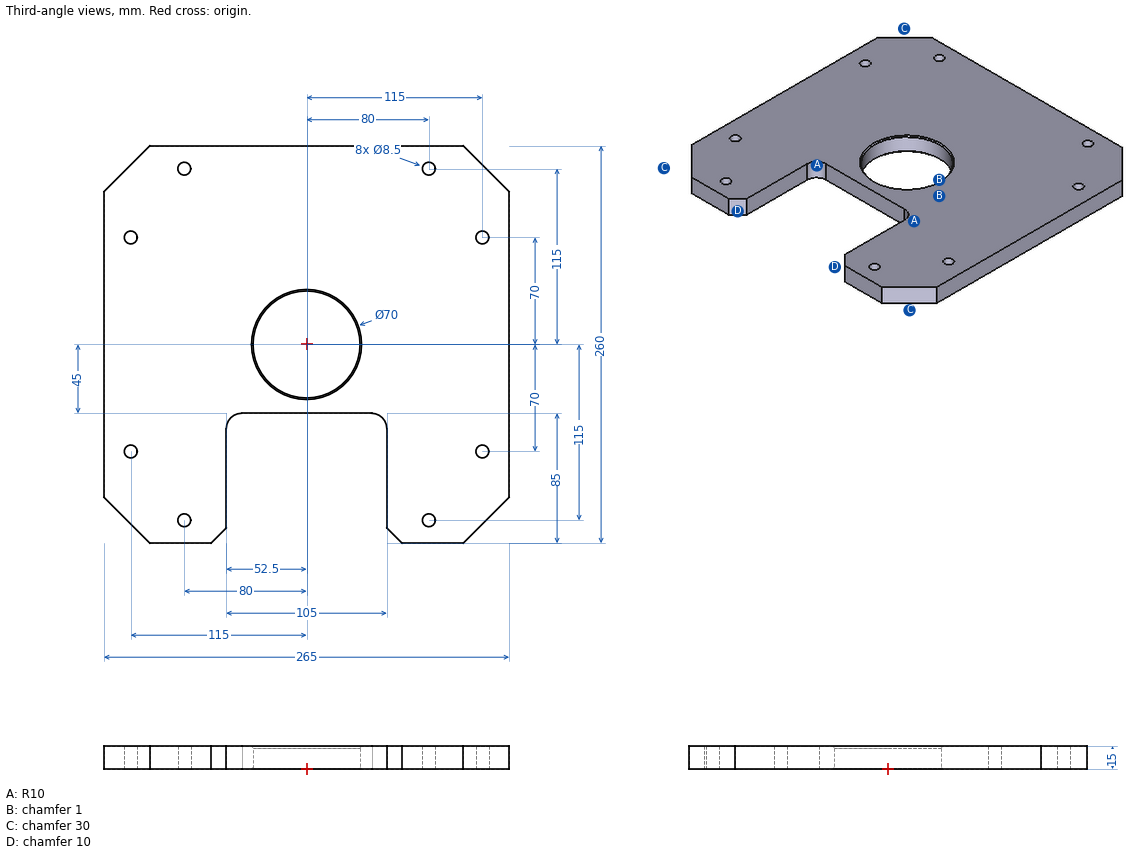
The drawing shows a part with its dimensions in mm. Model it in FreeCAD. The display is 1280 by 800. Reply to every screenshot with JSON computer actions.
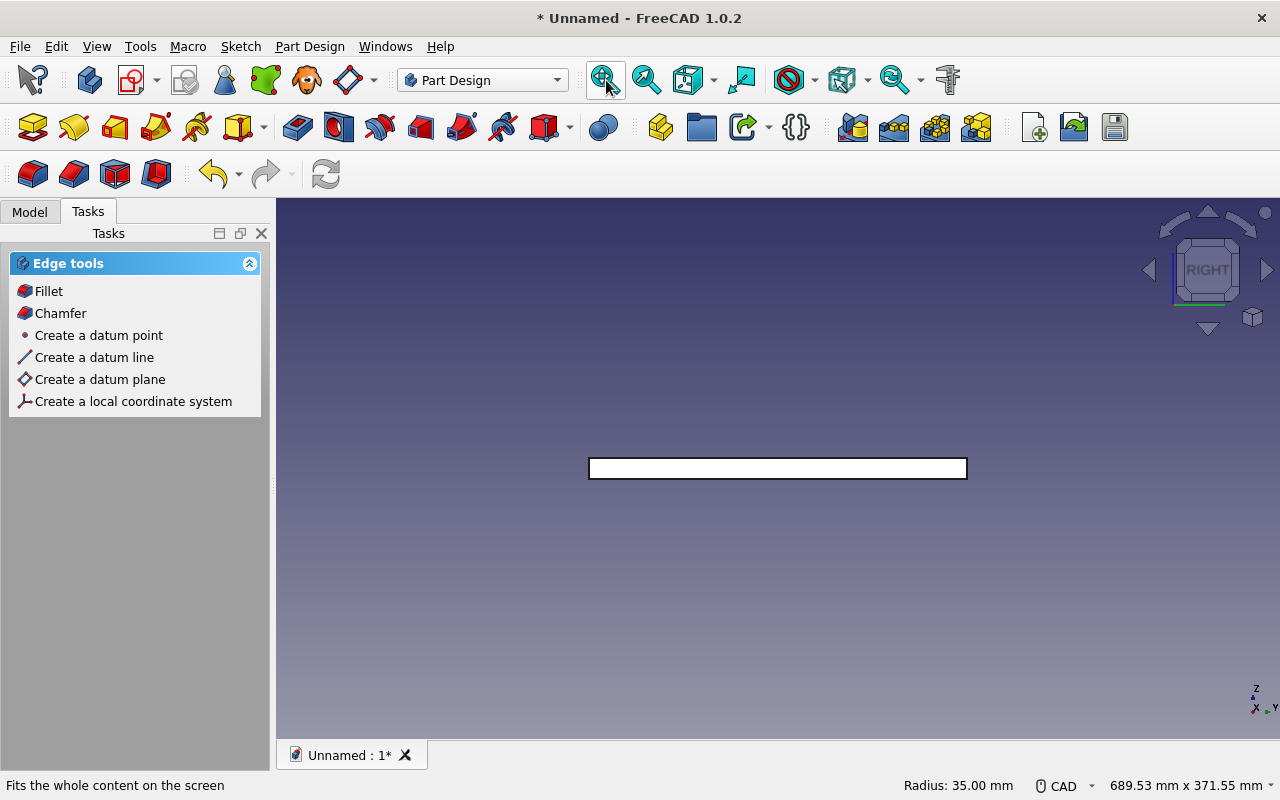
{"action": "key", "text": "5"}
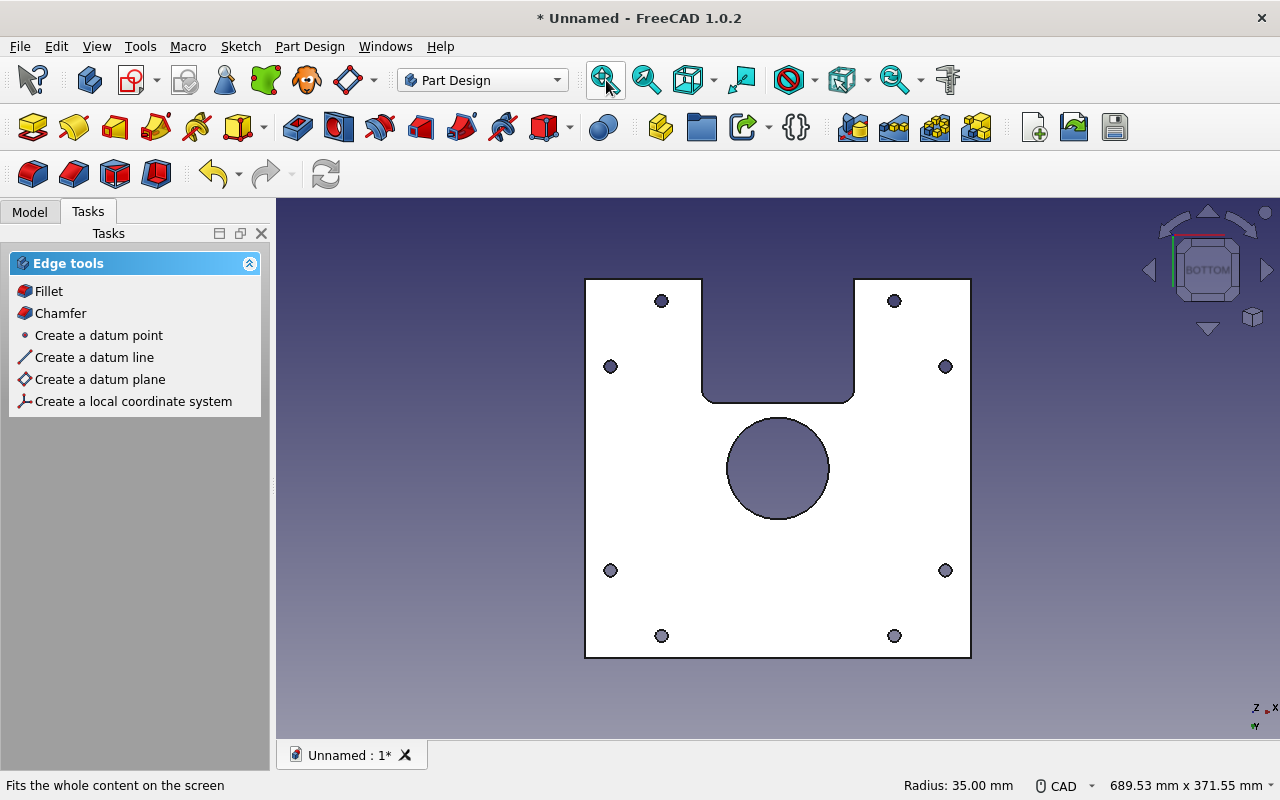
{"action": "left_click", "coordinate": [737, 497], "text": "ctrl"}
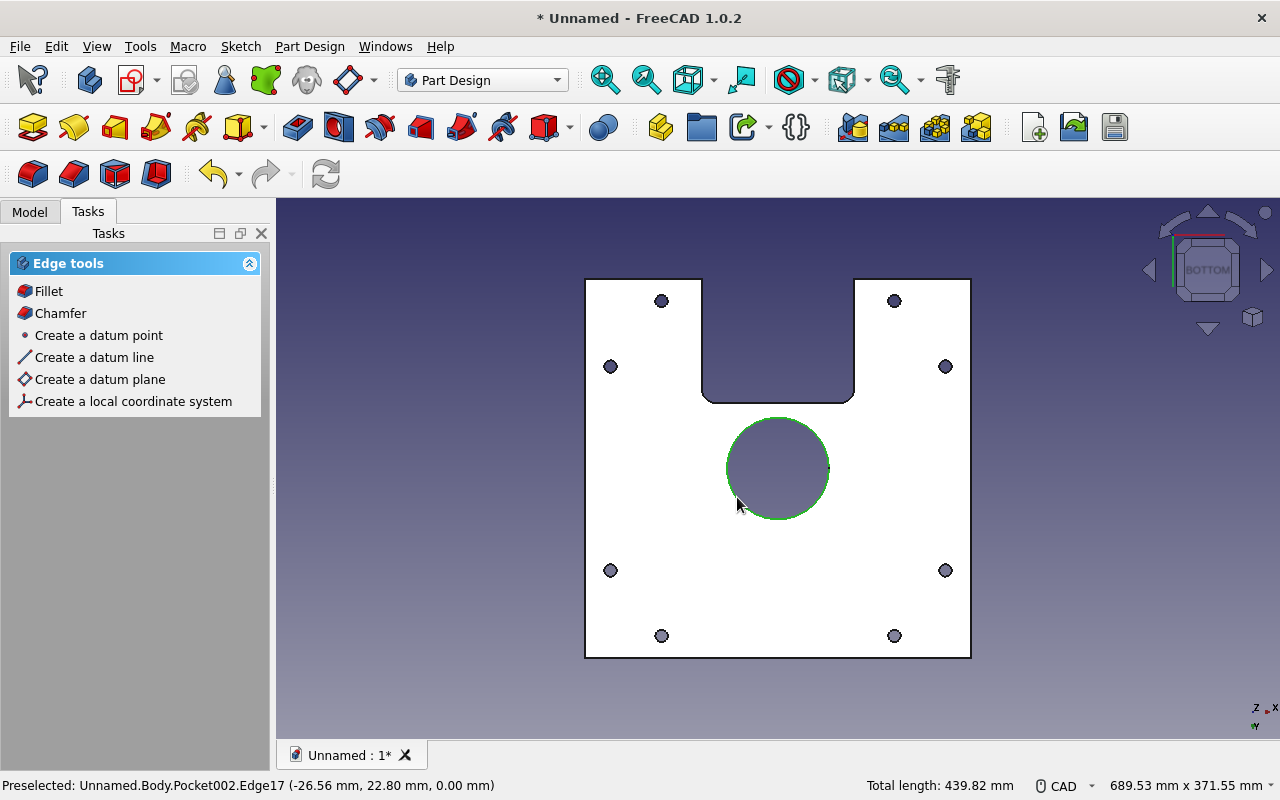
{"action": "left_click", "coordinate": [74, 174]}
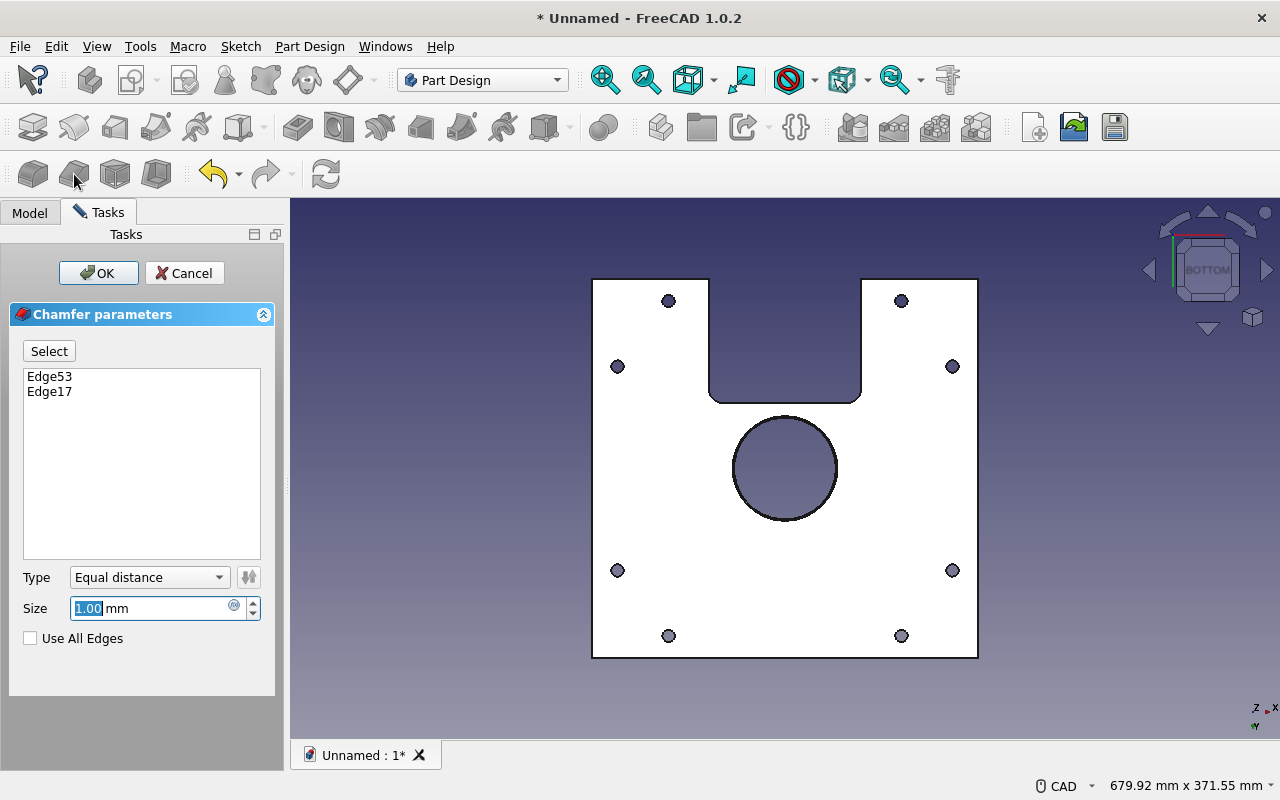
{"action": "type", "text": "1"}
{"action": "key", "text": "Tab"}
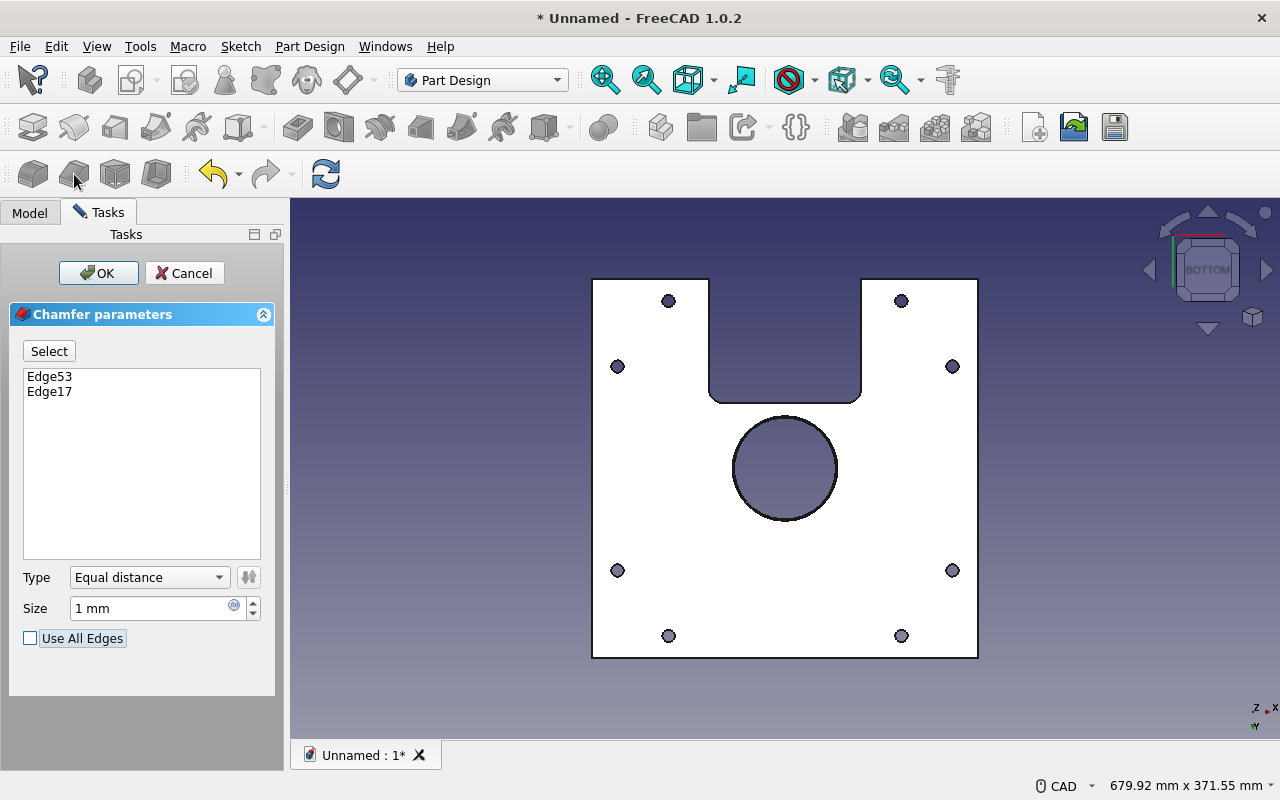
{"action": "left_click", "coordinate": [99, 273]}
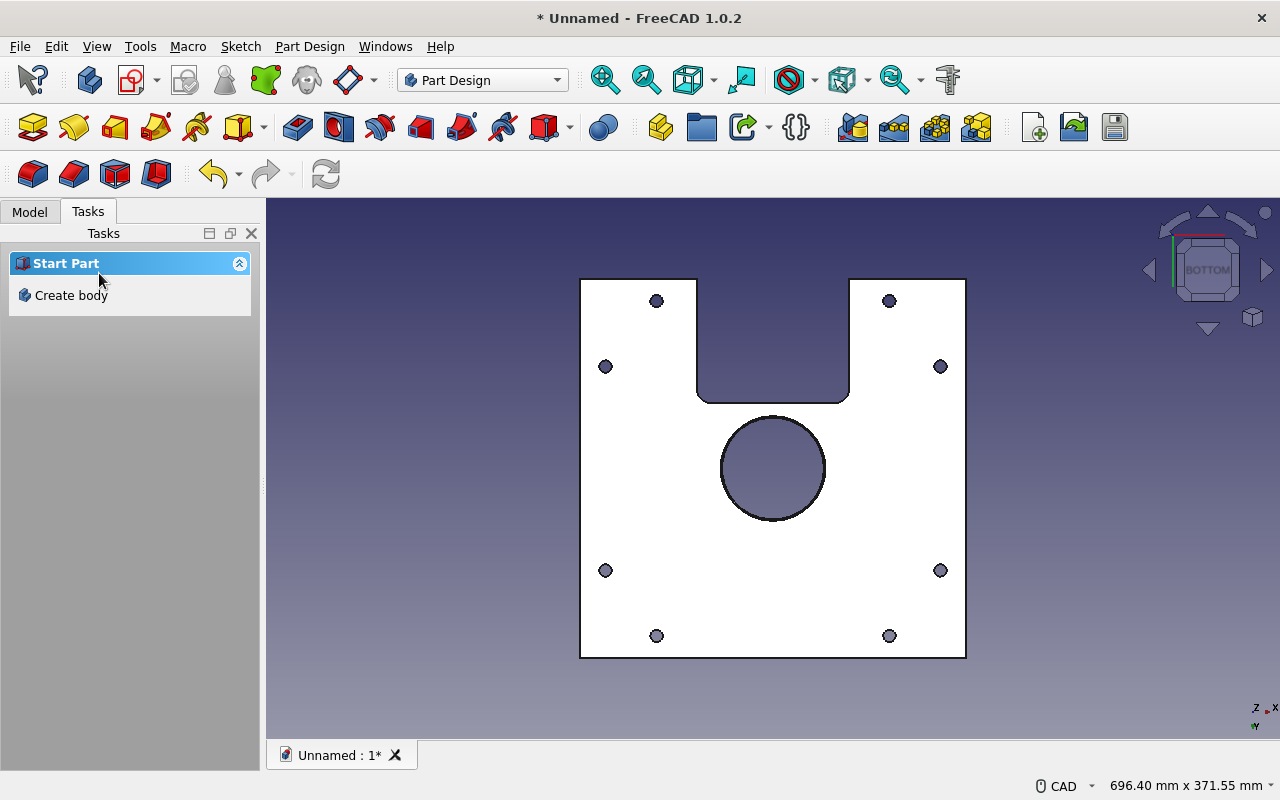
{"action": "scroll", "coordinate": [966, 278], "scroll_direction": "up", "scroll_amount": 4}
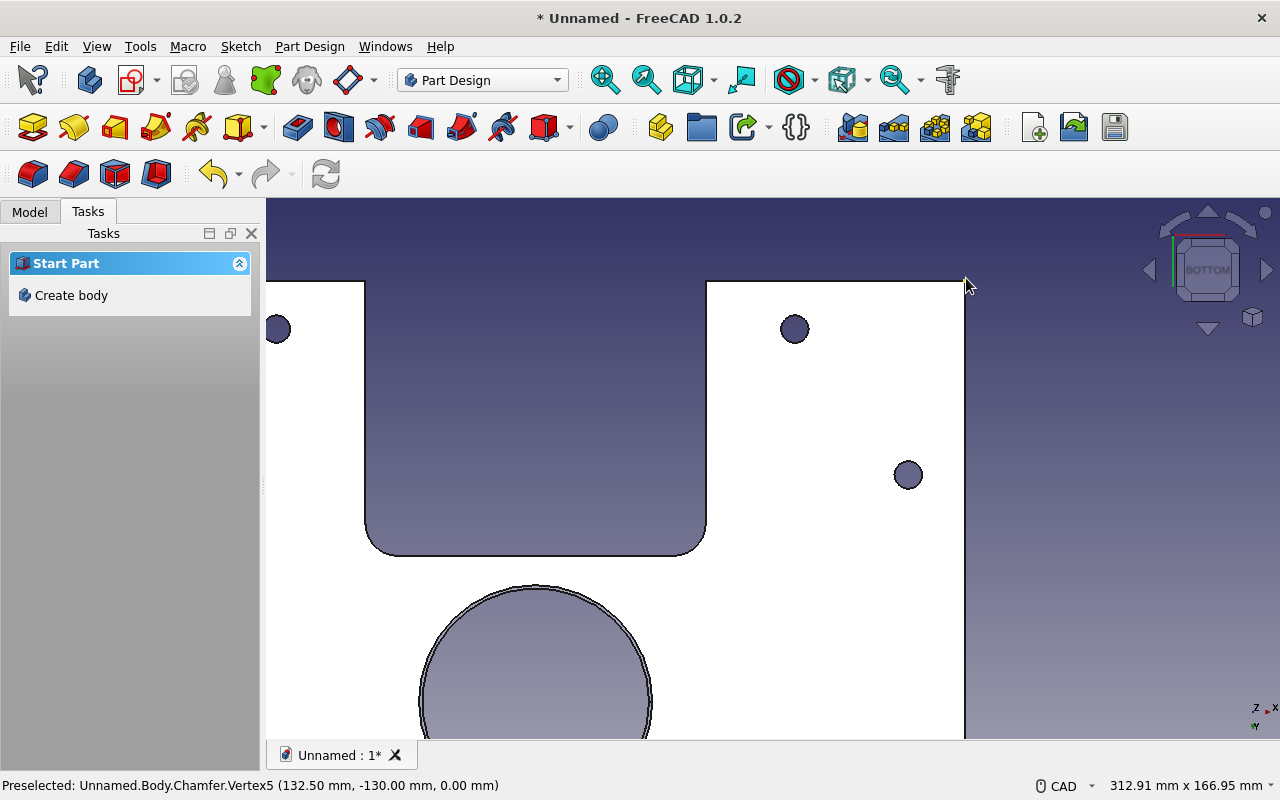
{"action": "key", "text": "v f"}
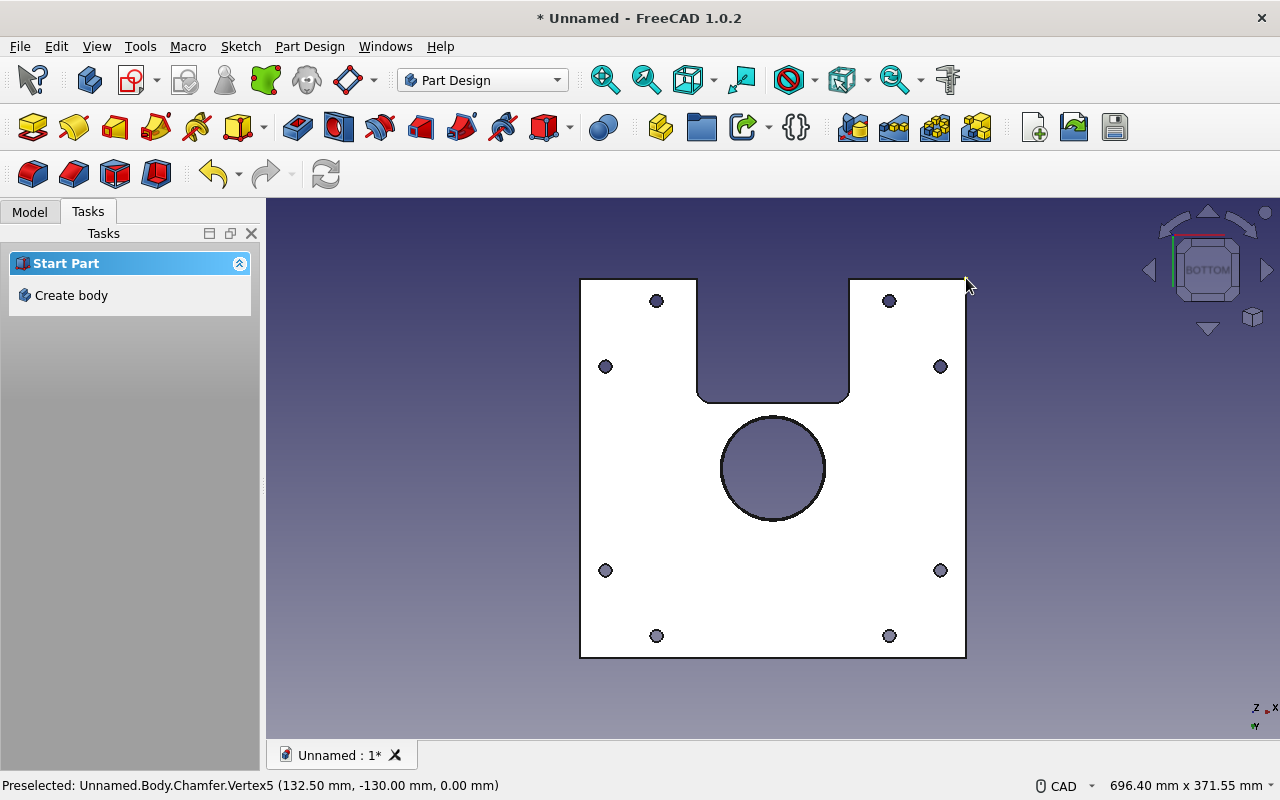
{"action": "key", "text": "0"}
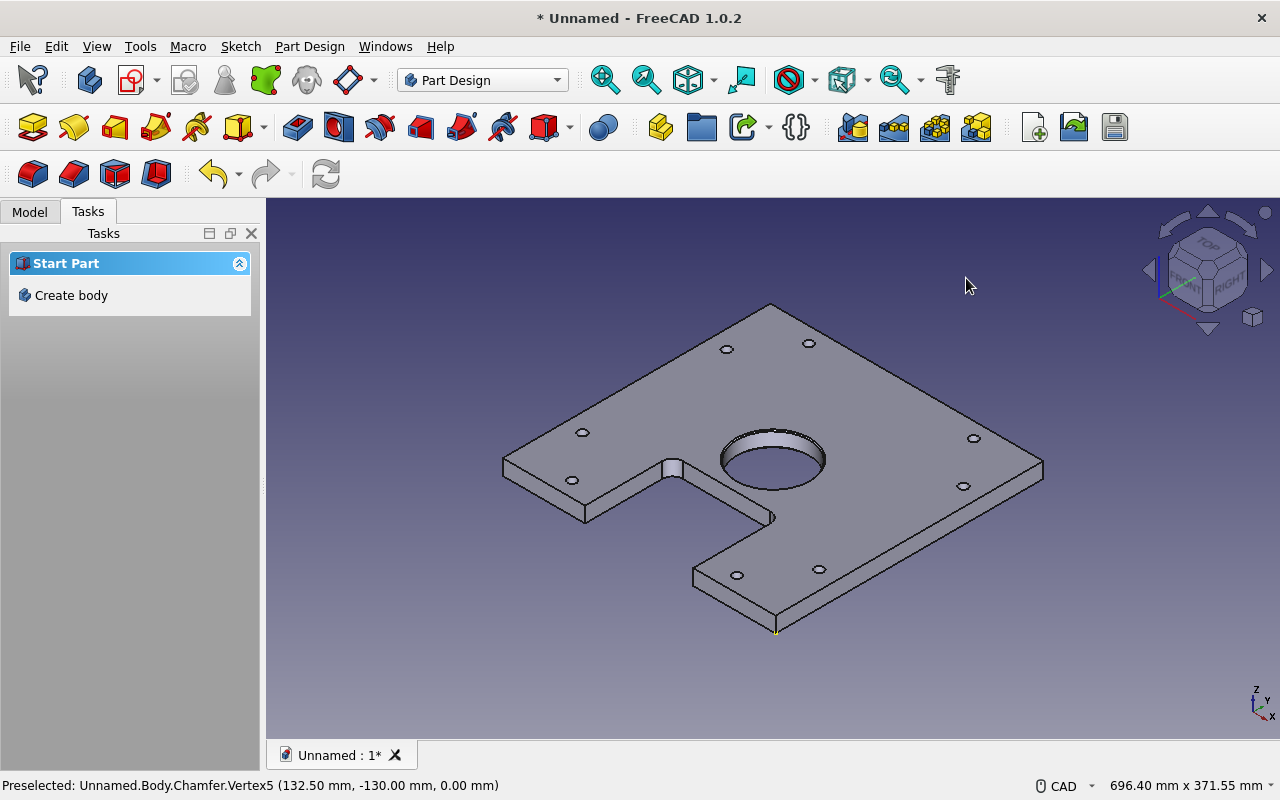
{"action": "left_click", "coordinate": [776, 624]}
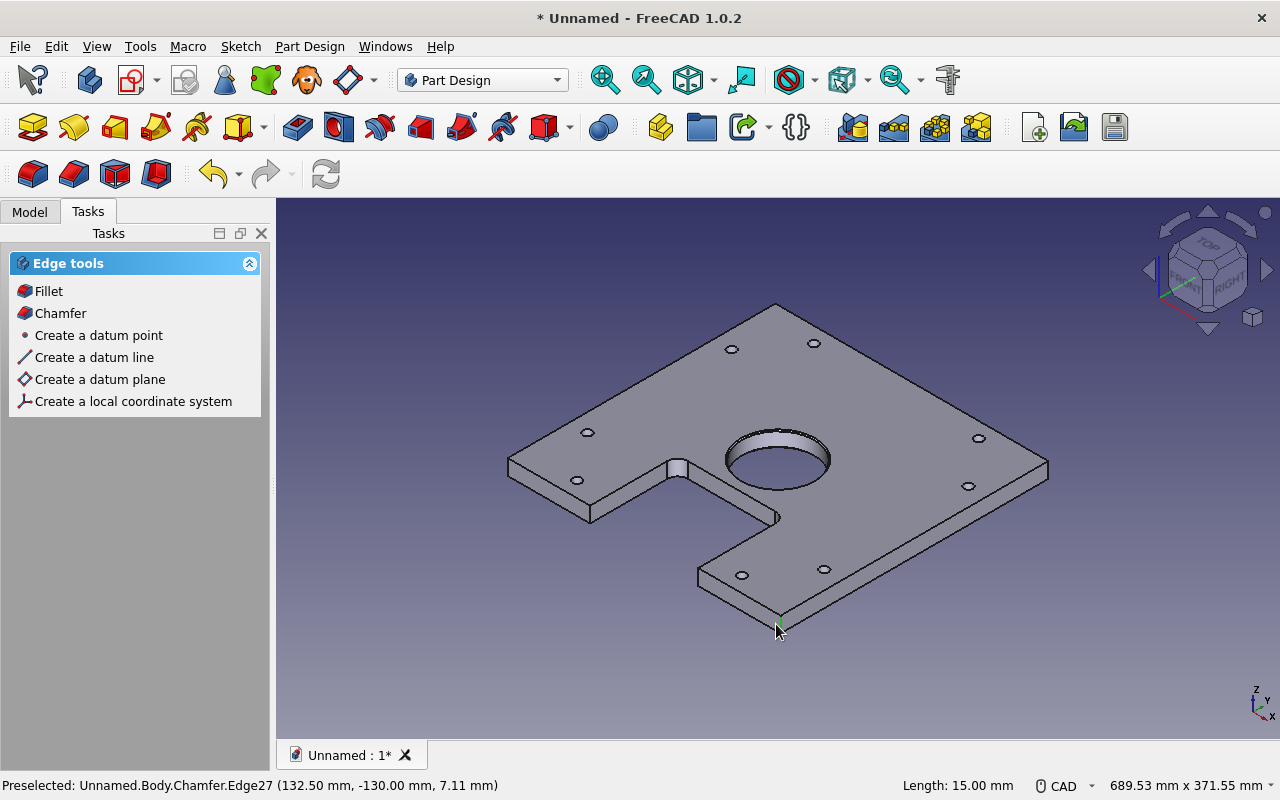
{"action": "scroll", "coordinate": [508, 466], "scroll_direction": "up", "scroll_amount": 4}